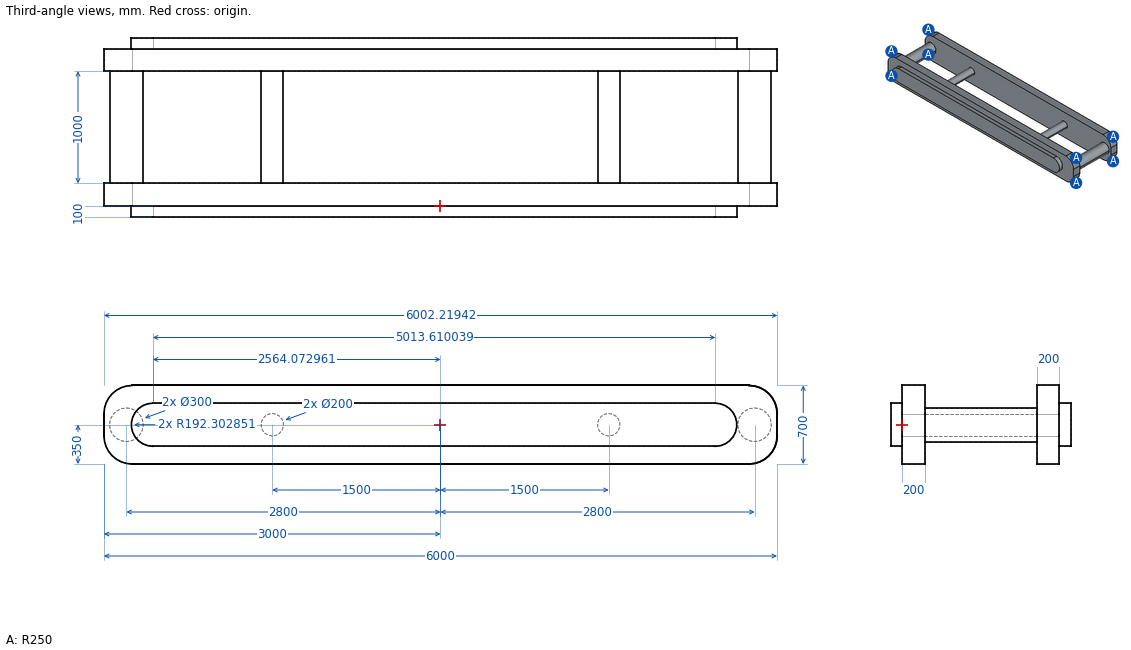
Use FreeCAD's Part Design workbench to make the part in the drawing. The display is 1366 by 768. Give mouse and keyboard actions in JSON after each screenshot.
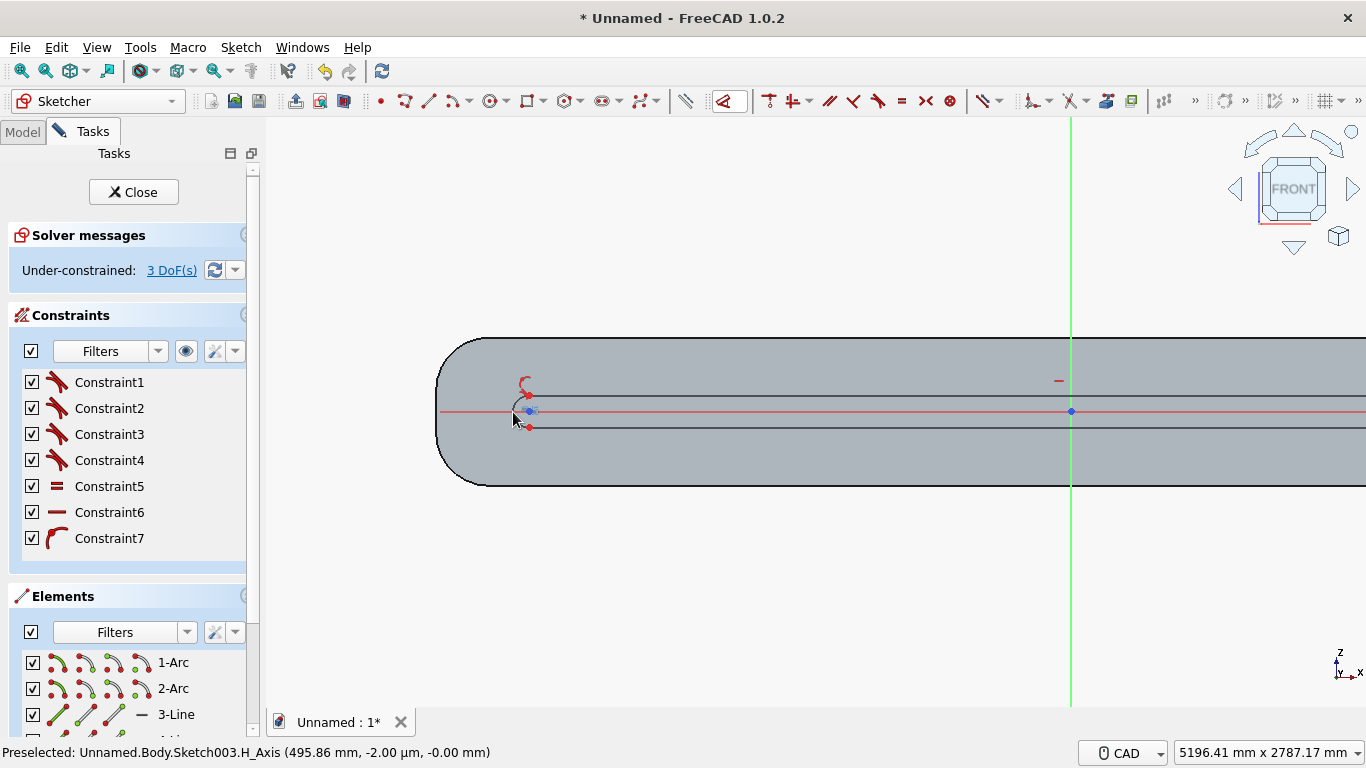
{"action": "left_click", "coordinate": [513, 412]}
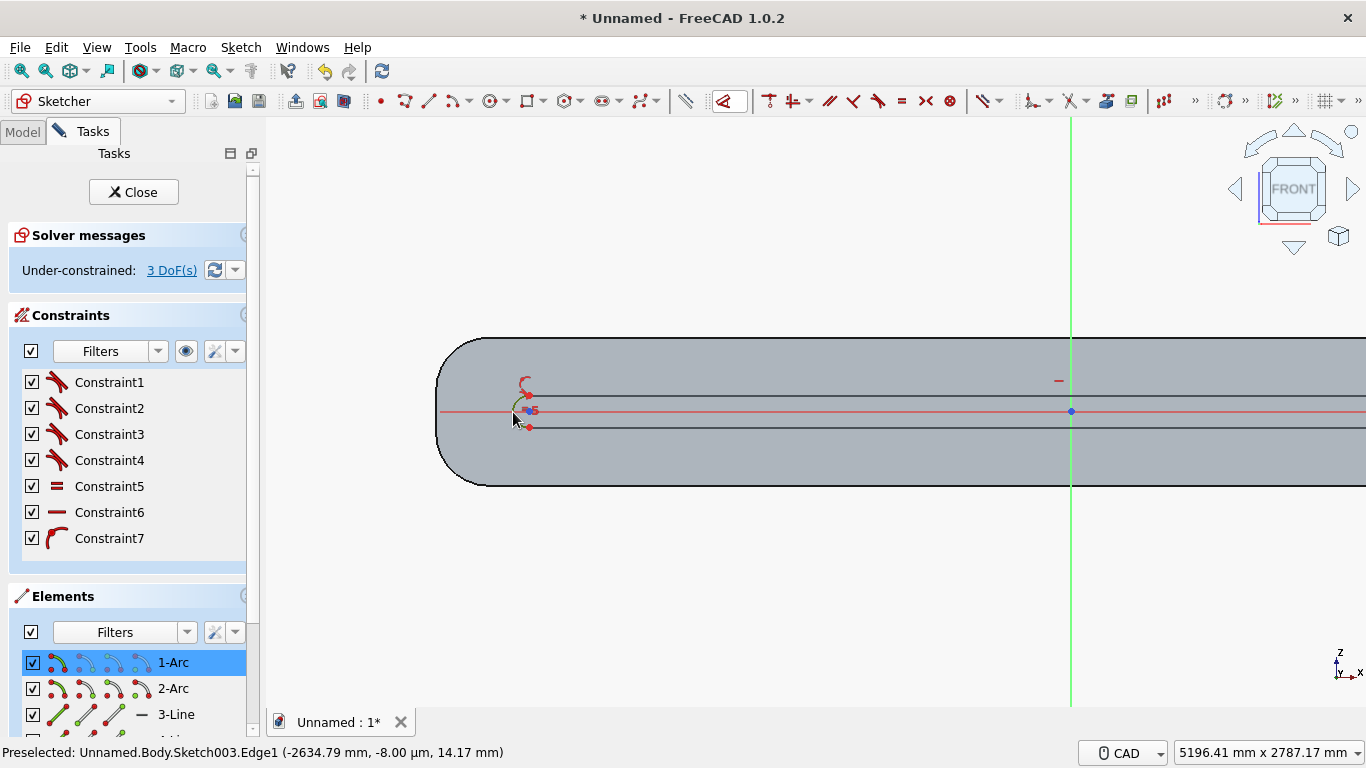
{"action": "key", "text": "k r"}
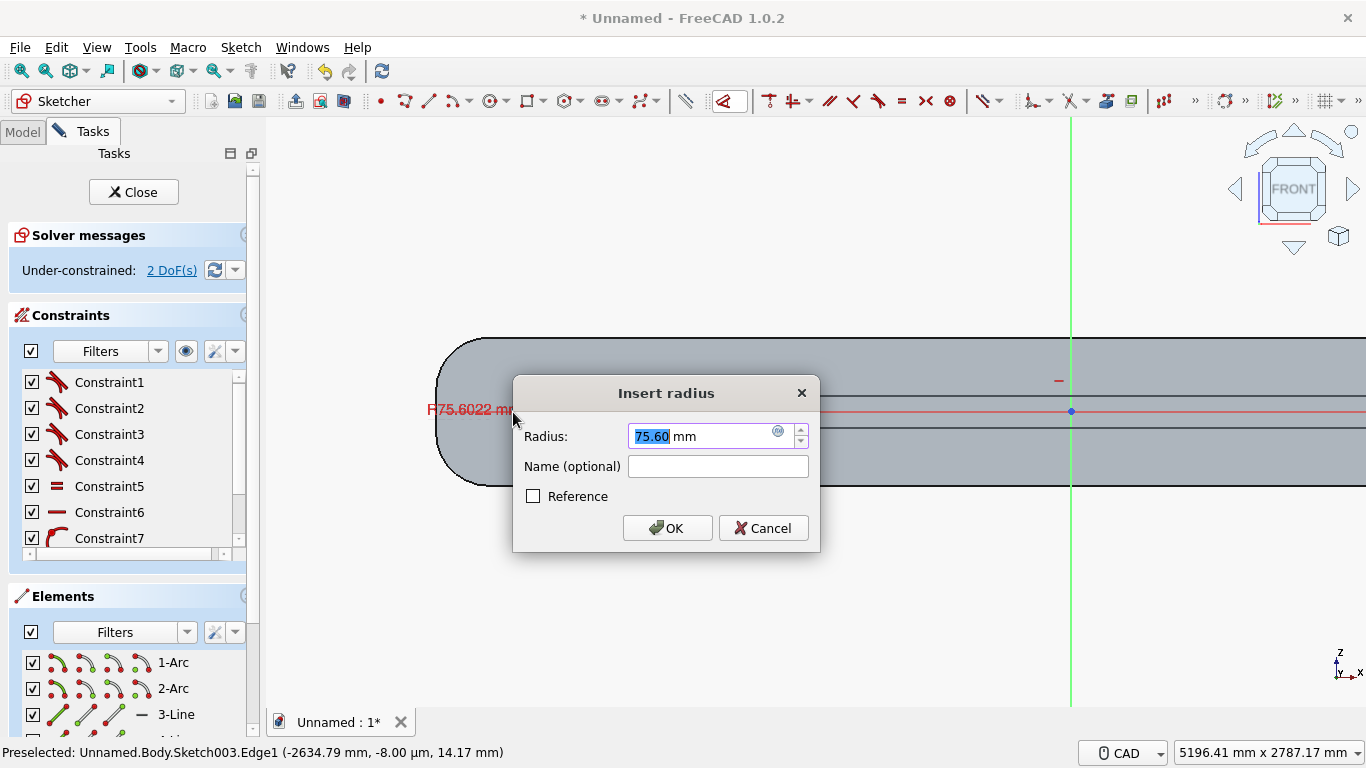
{"action": "type", "text": "192.302851"}
{"action": "key", "text": "Return"}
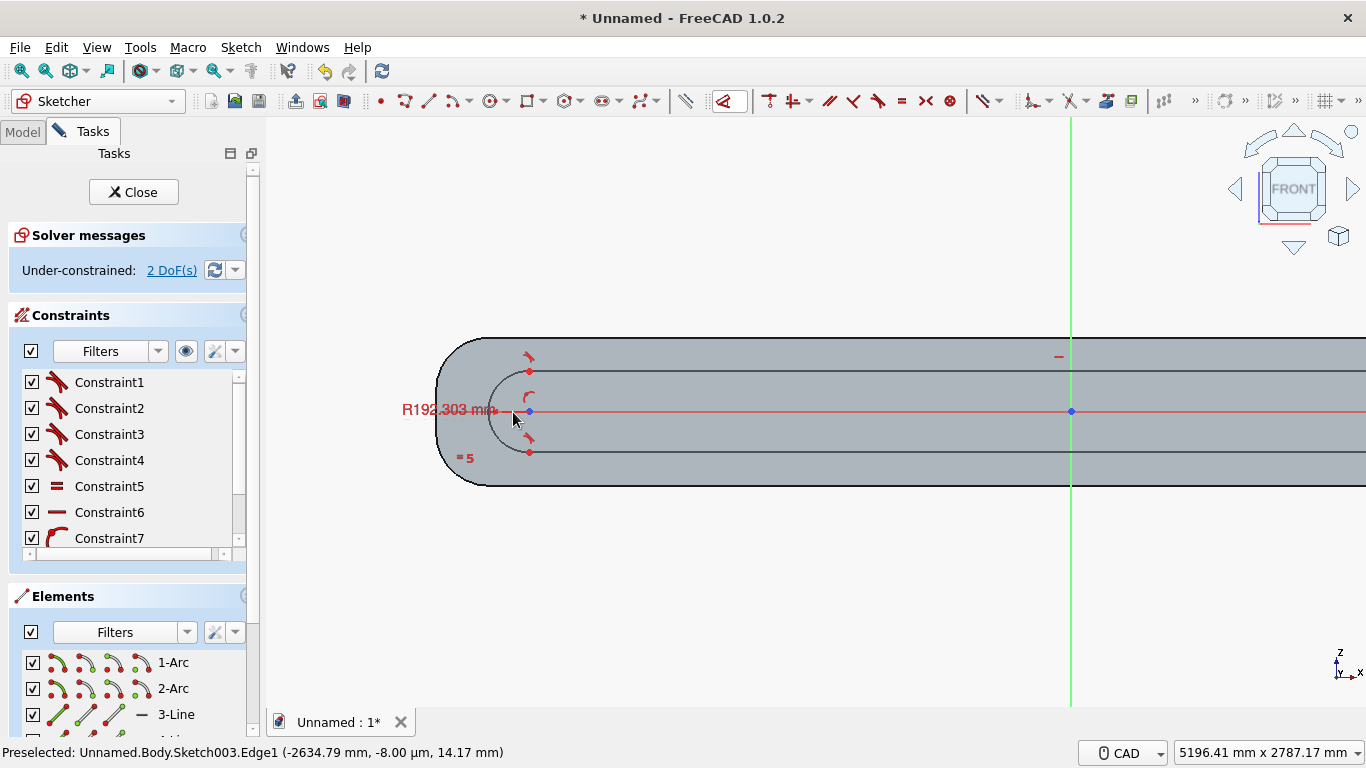
{"action": "left_click", "coordinate": [847, 371]}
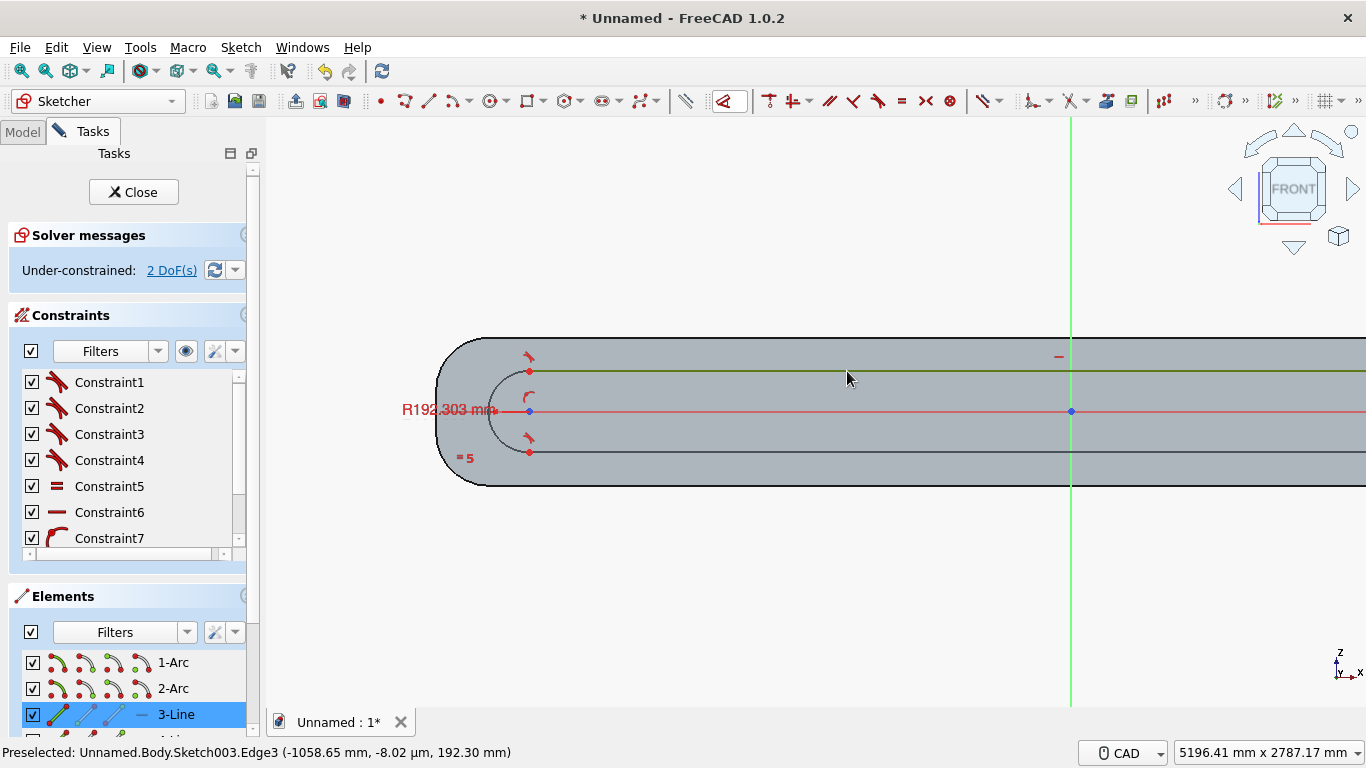
{"action": "key", "text": "l"}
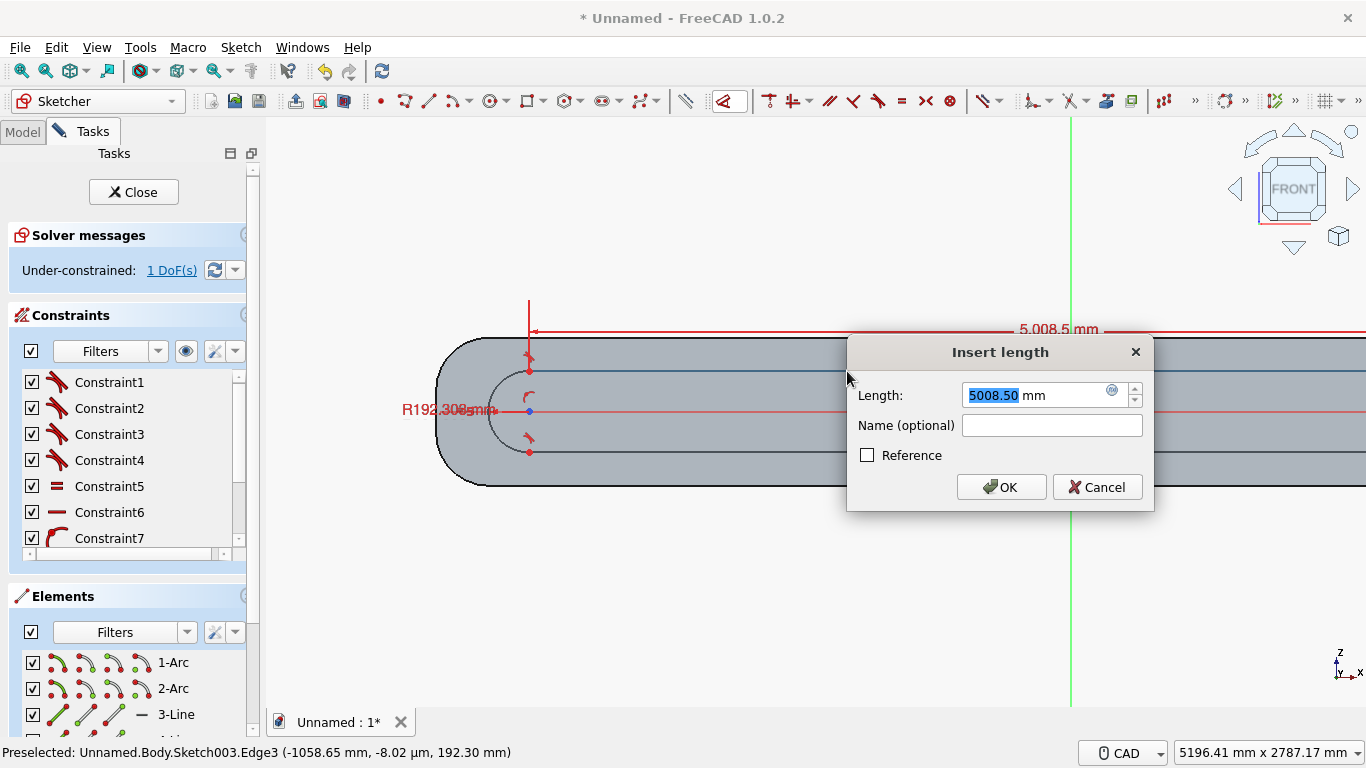
{"action": "type", "text": "5013.610039"}
{"action": "key", "text": "Return"}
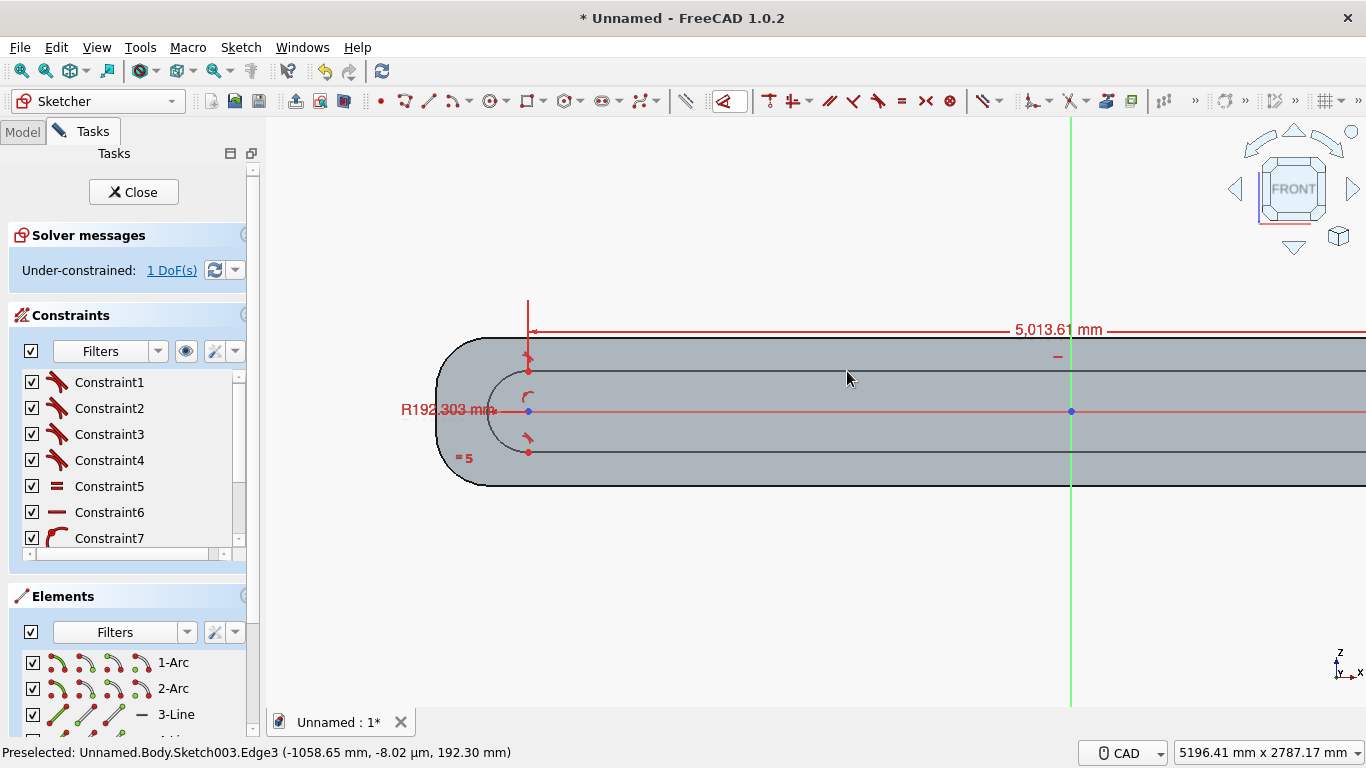
{"action": "left_click", "coordinate": [528, 371]}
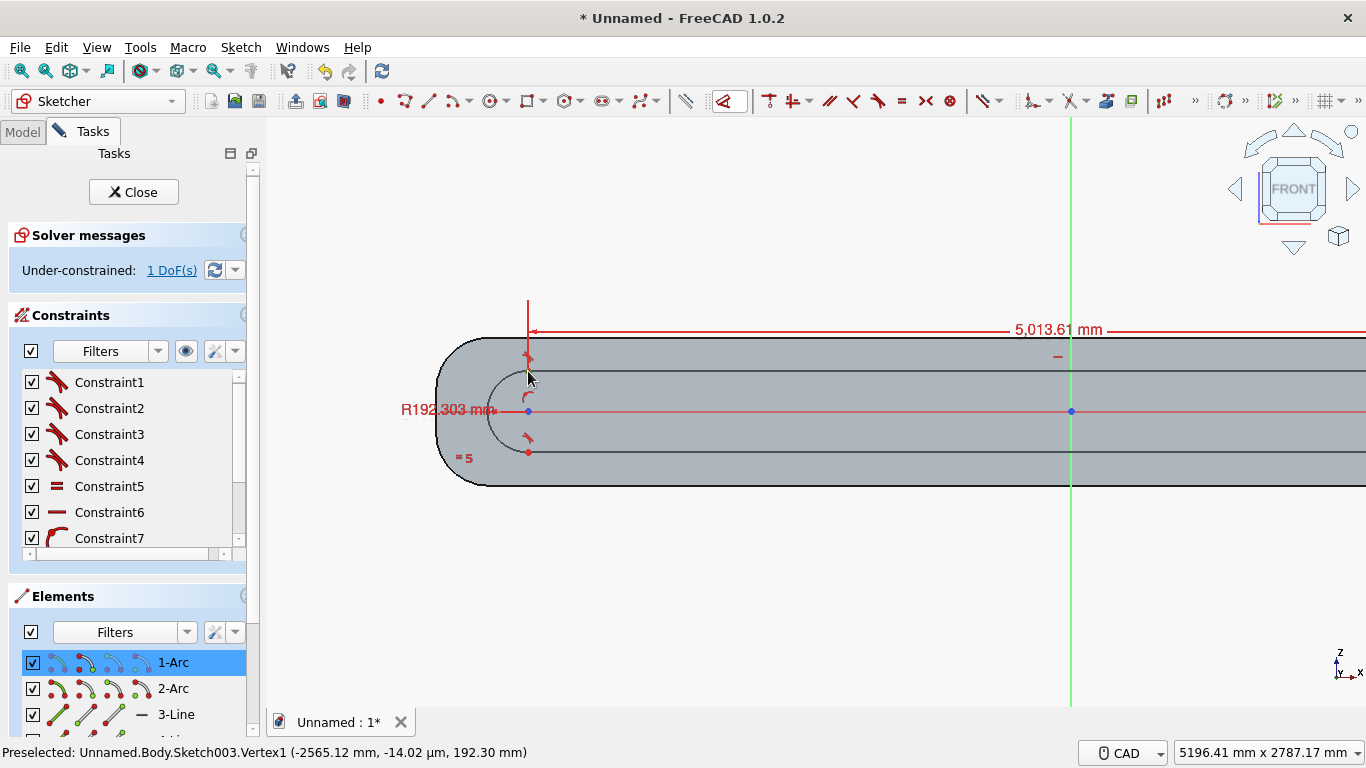
{"action": "left_click", "coordinate": [742, 102]}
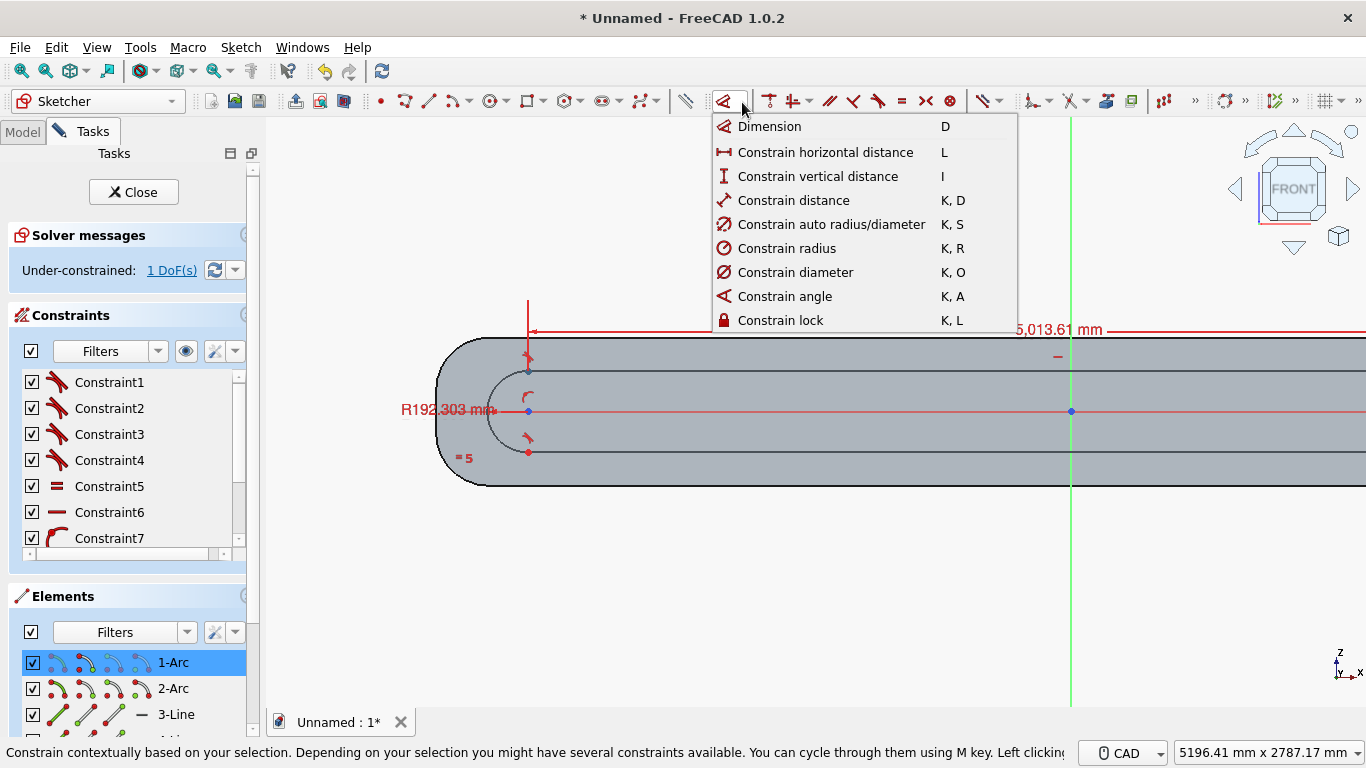
{"action": "left_click", "coordinate": [865, 152]}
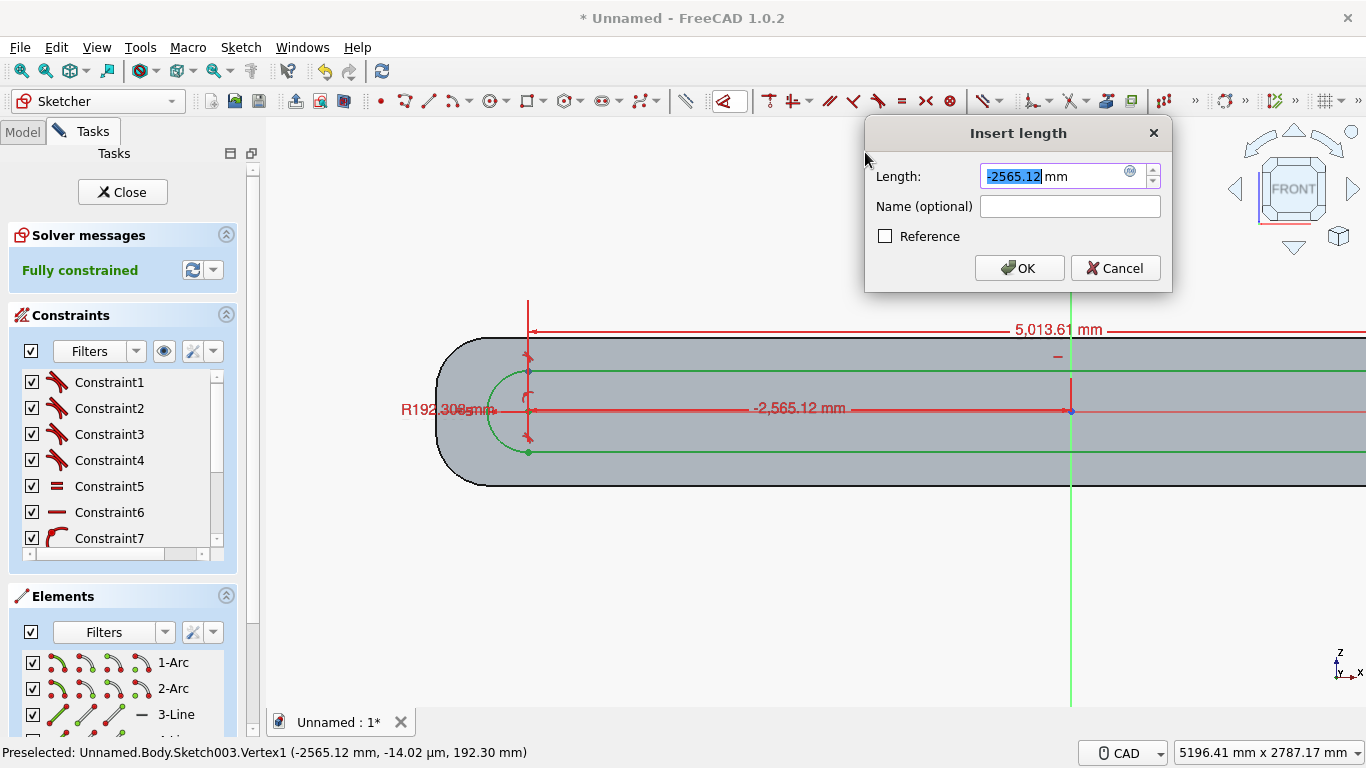
{"action": "type", "text": "-2564.072961"}
{"action": "key", "text": "Return"}